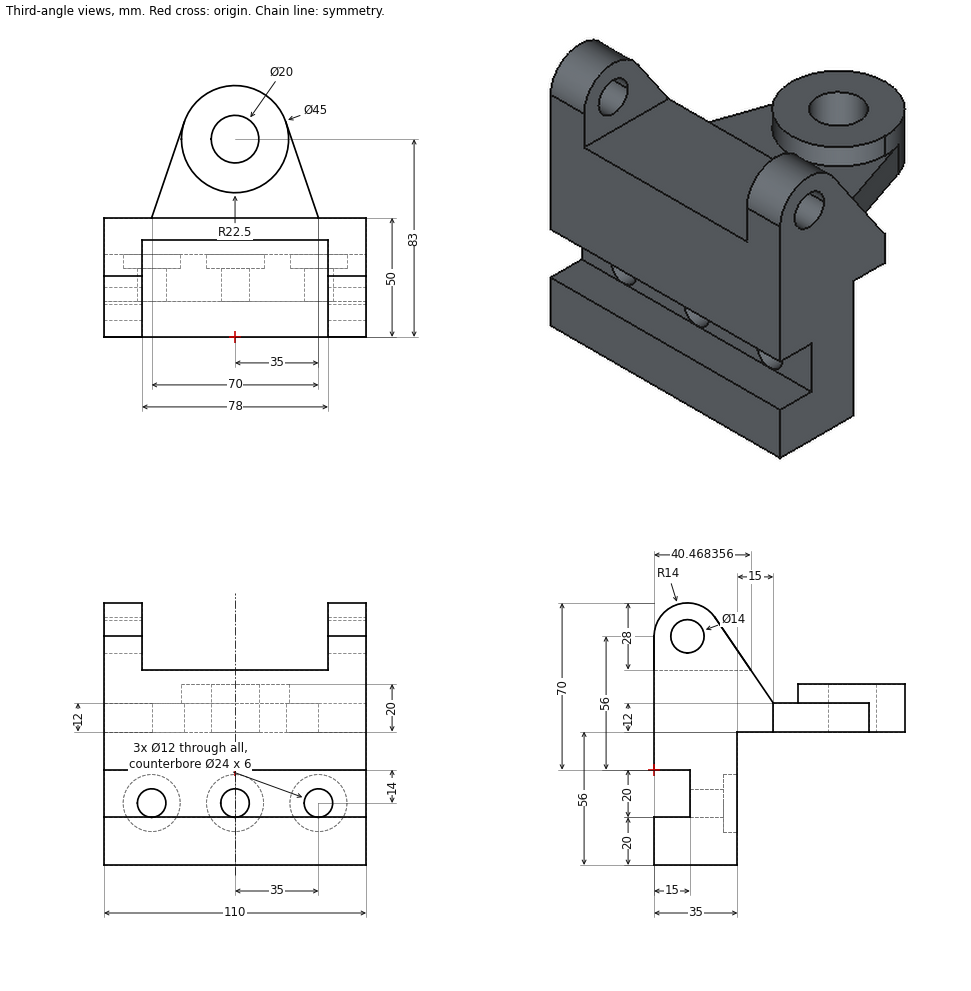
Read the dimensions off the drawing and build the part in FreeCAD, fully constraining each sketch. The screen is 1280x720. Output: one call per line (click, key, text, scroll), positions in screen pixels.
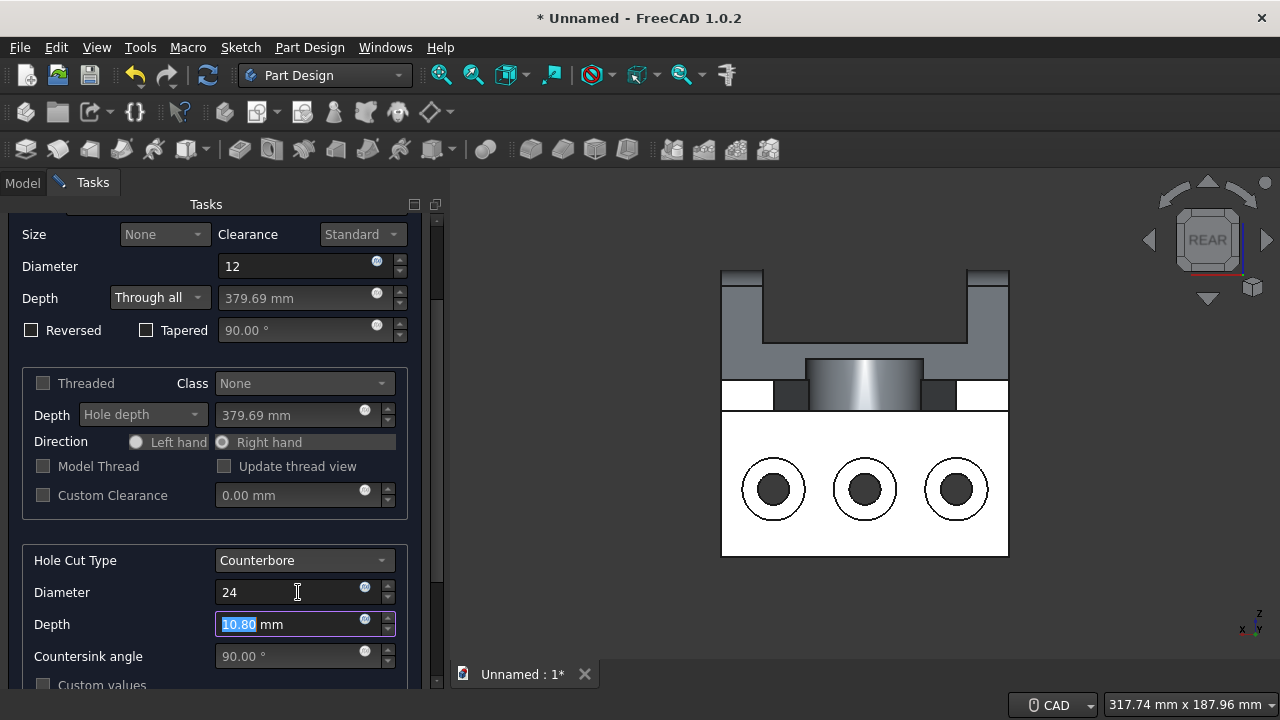
text(6)
key(Tab)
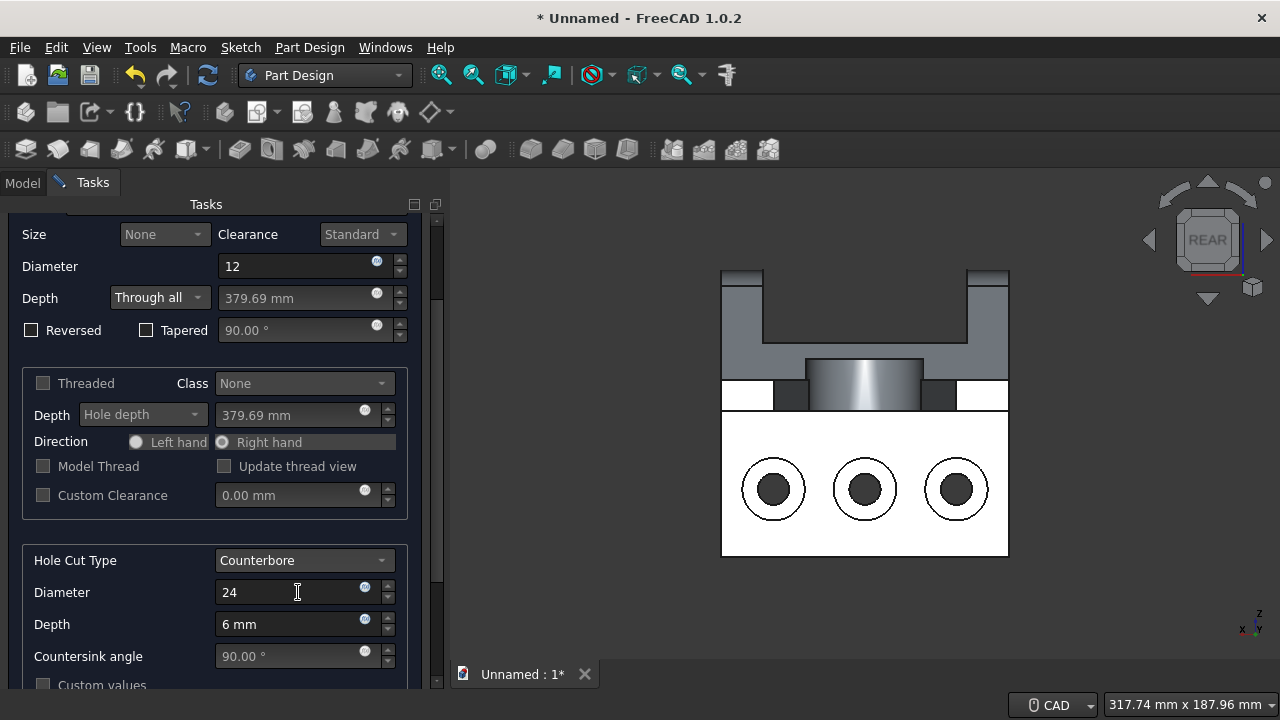
scroll(437, 451, up, 3)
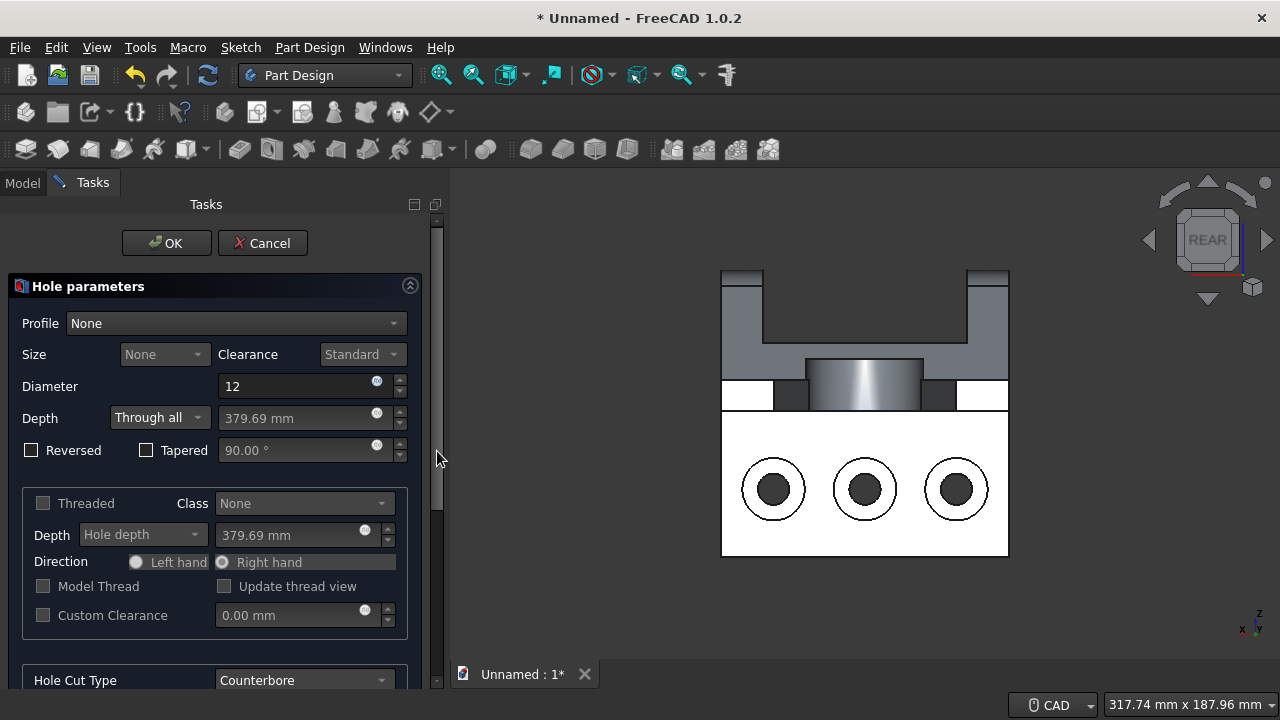
click(167, 243)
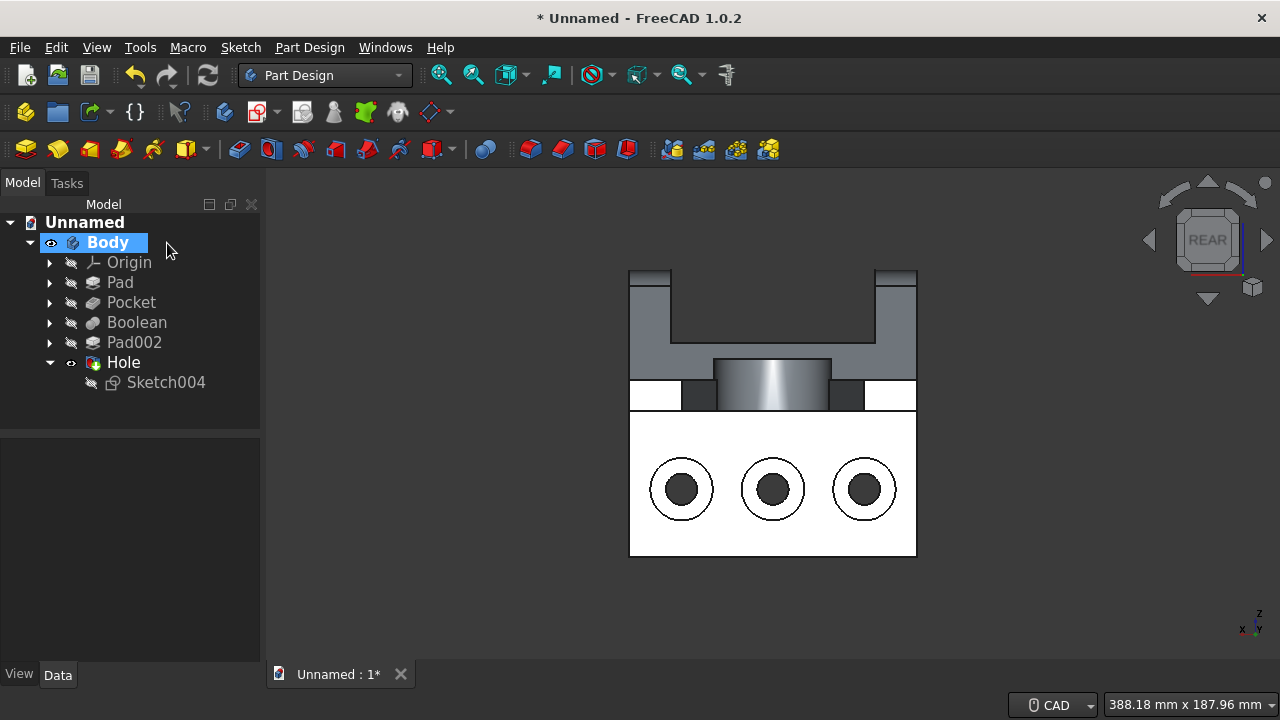
key(0)